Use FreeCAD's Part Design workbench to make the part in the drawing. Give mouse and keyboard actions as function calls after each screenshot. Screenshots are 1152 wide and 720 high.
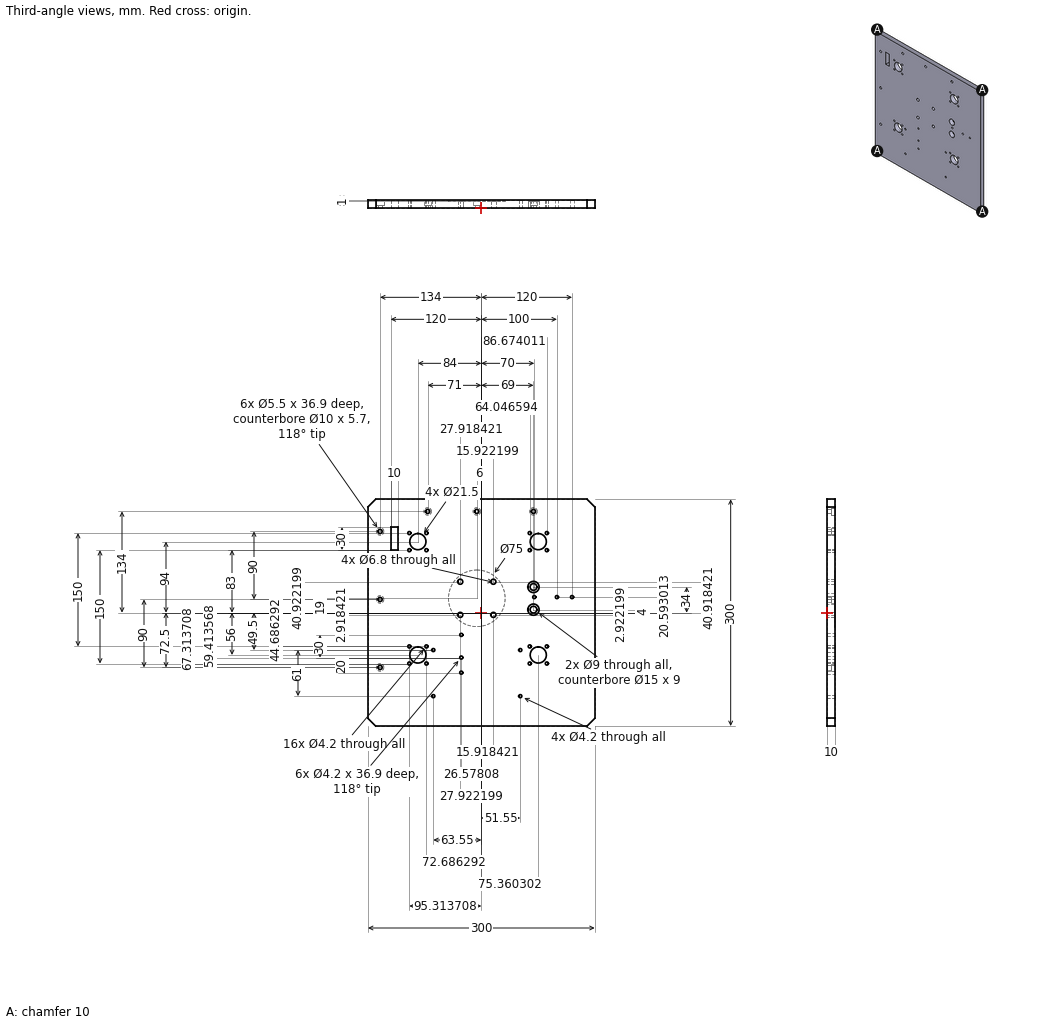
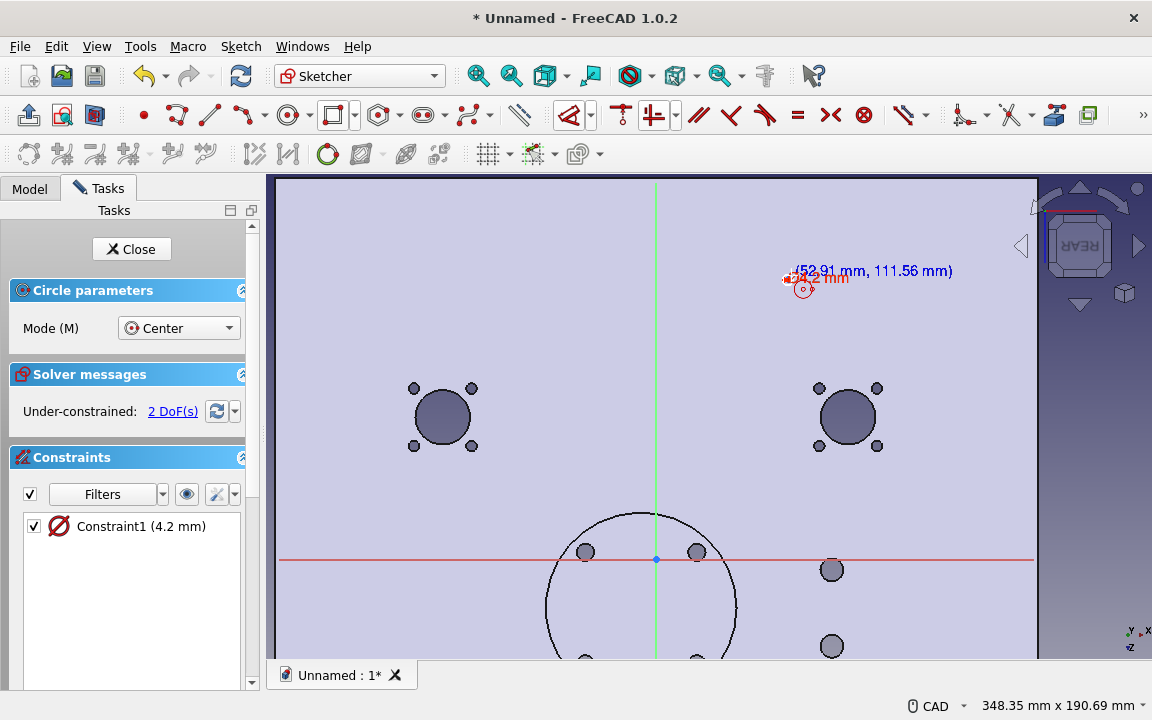
scroll(495, 279, up, 8)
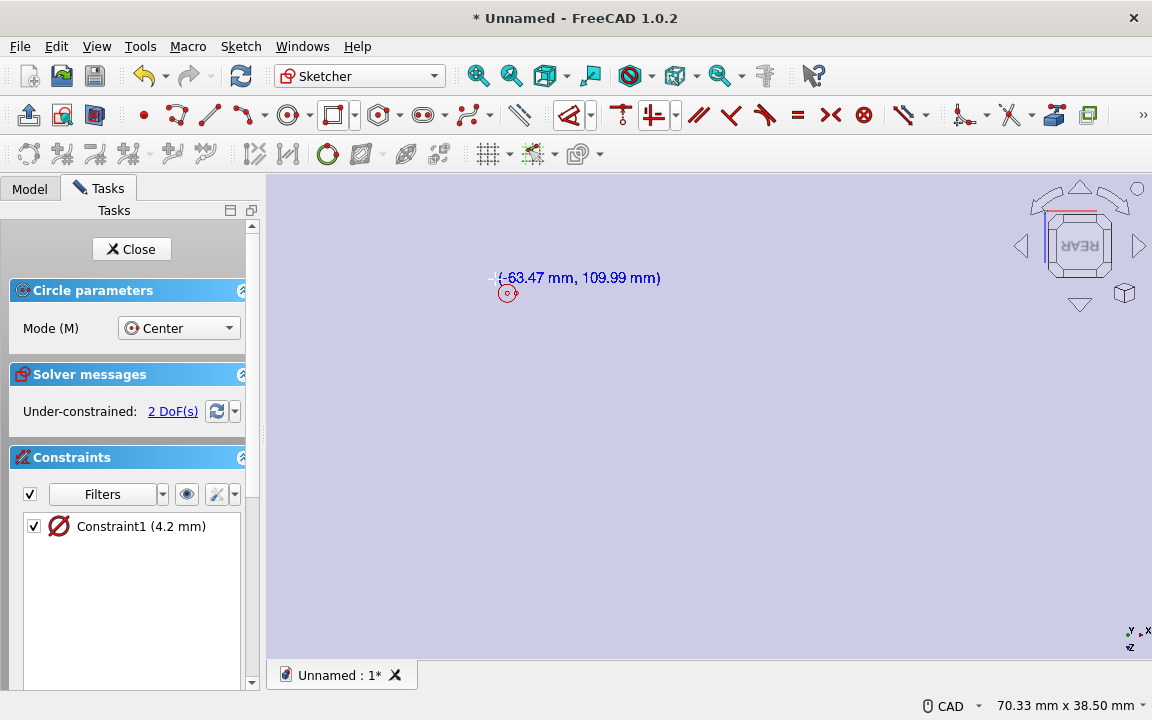
scroll(494, 279, down, 8)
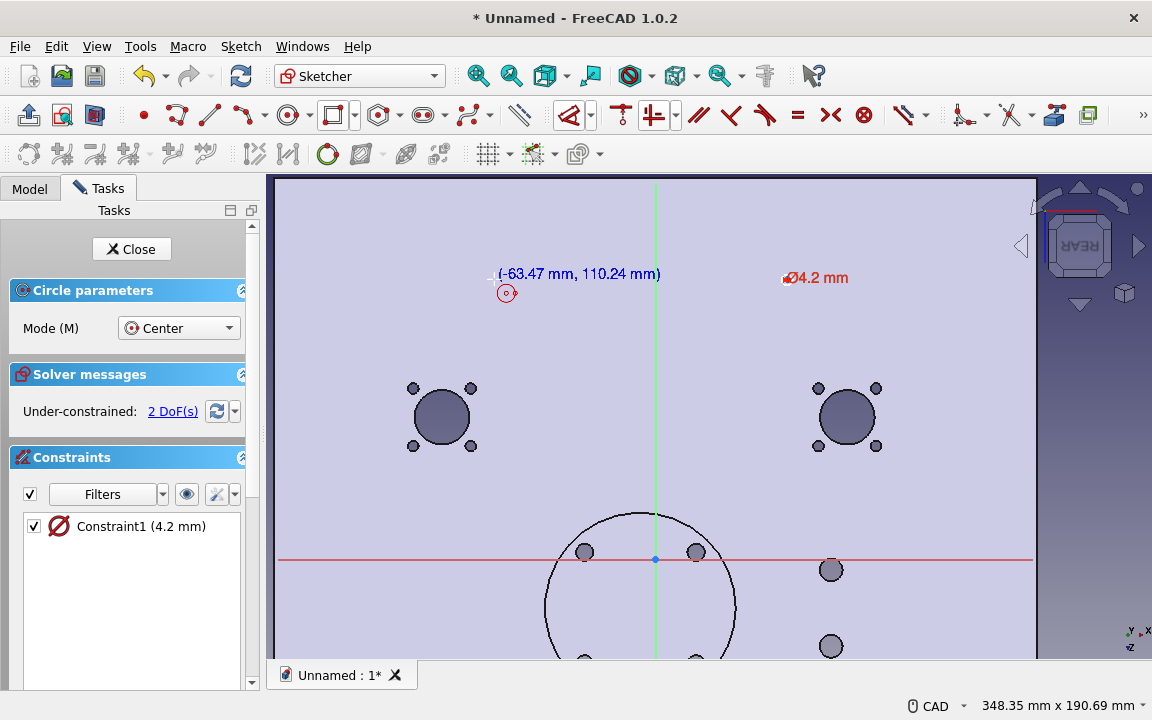
click(494, 279)
move(498, 275)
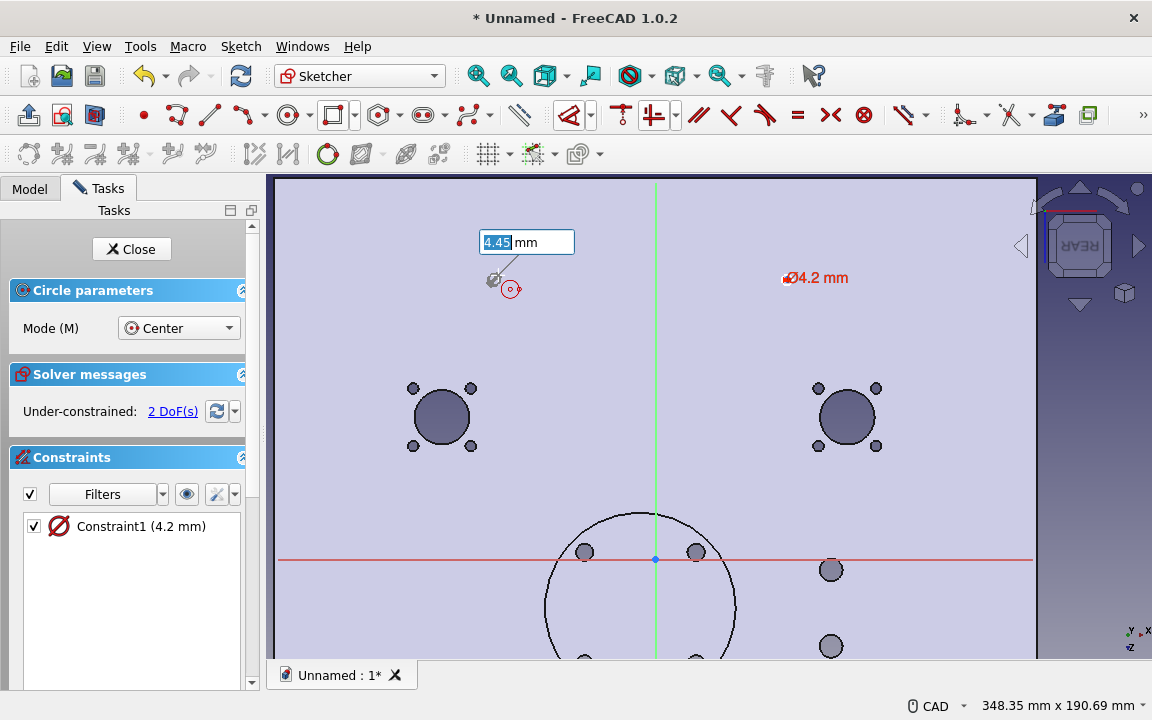
text(4.2)
key(Return)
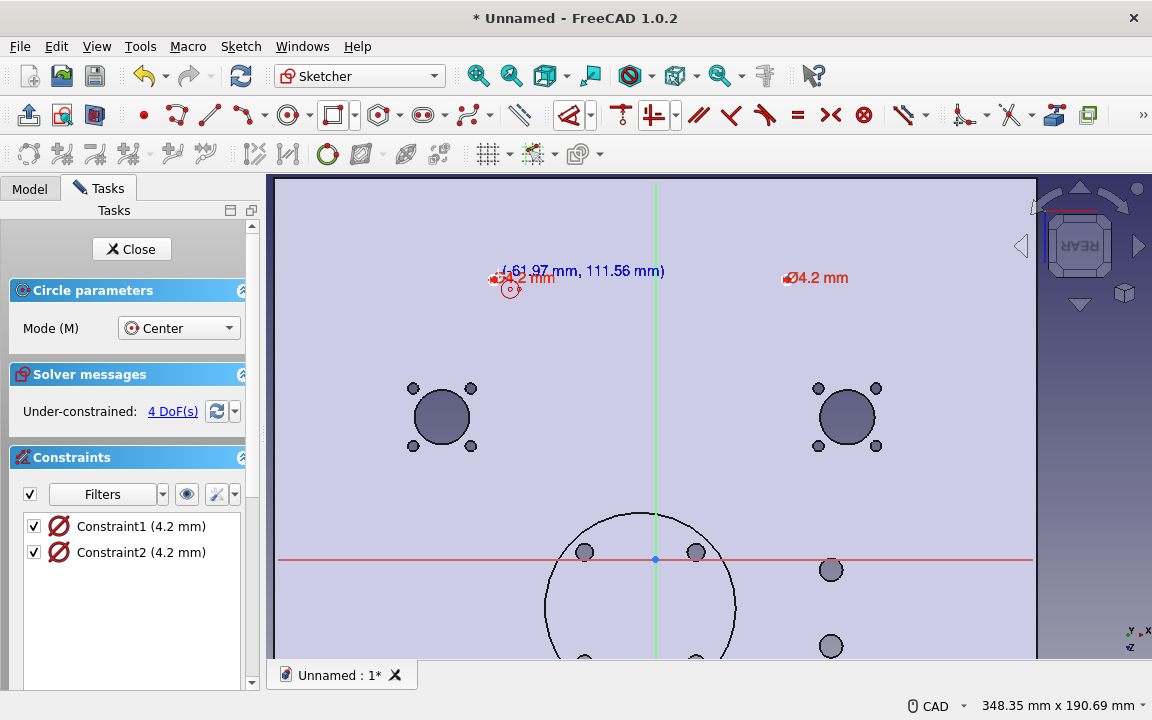
scroll(494, 434, up, 8)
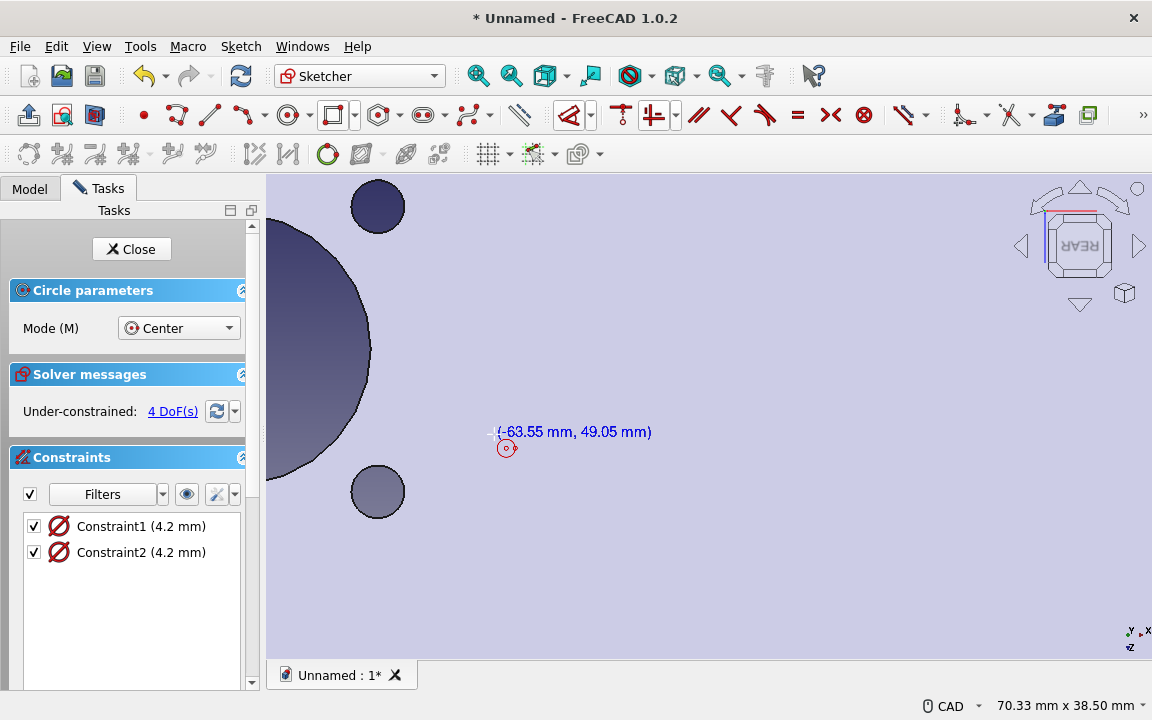
scroll(494, 434, down, 8)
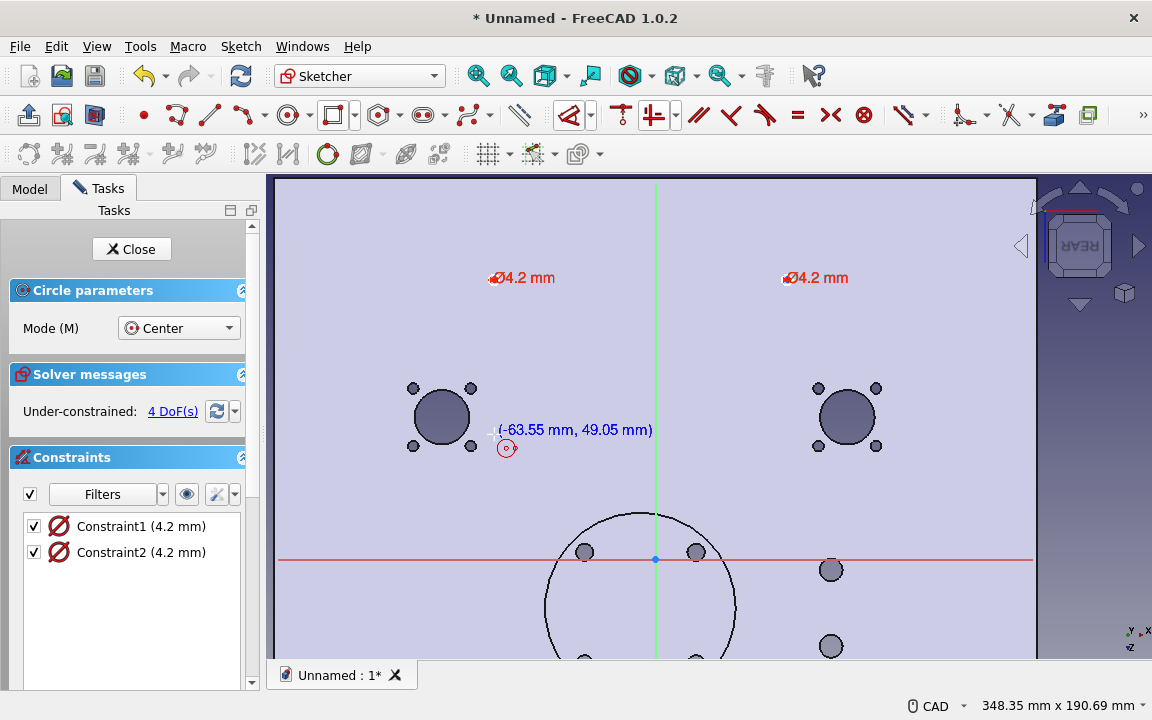
click(494, 434)
move(498, 430)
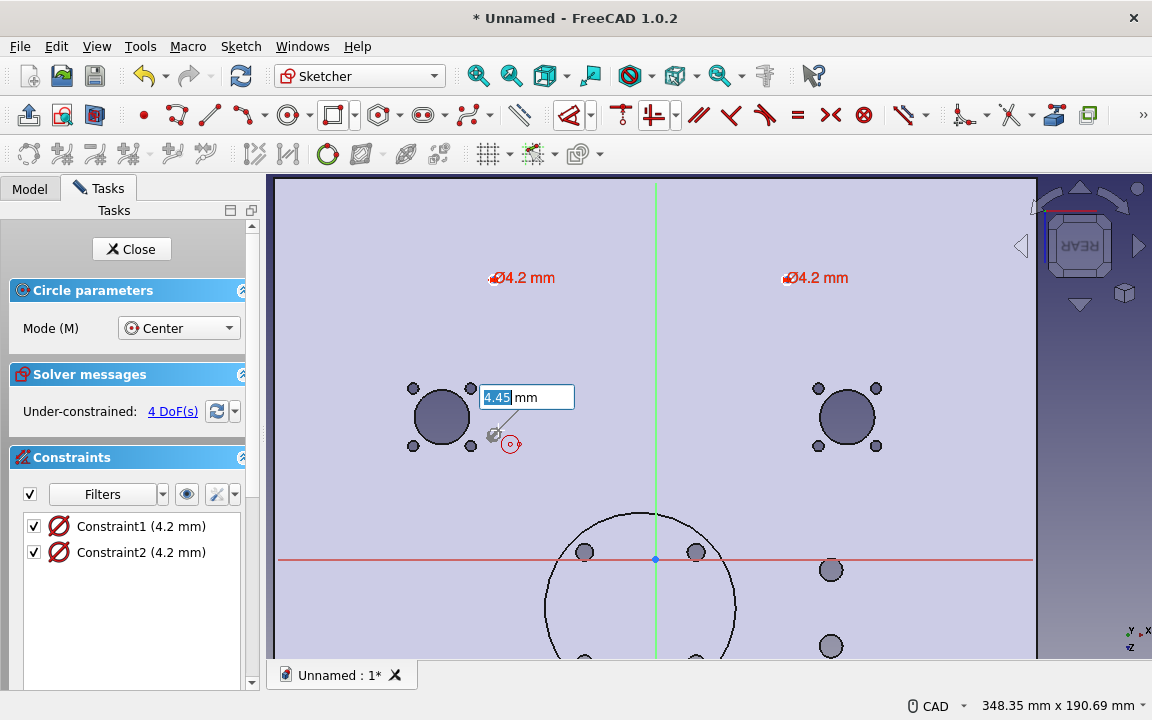
text(4.2)
key(Return)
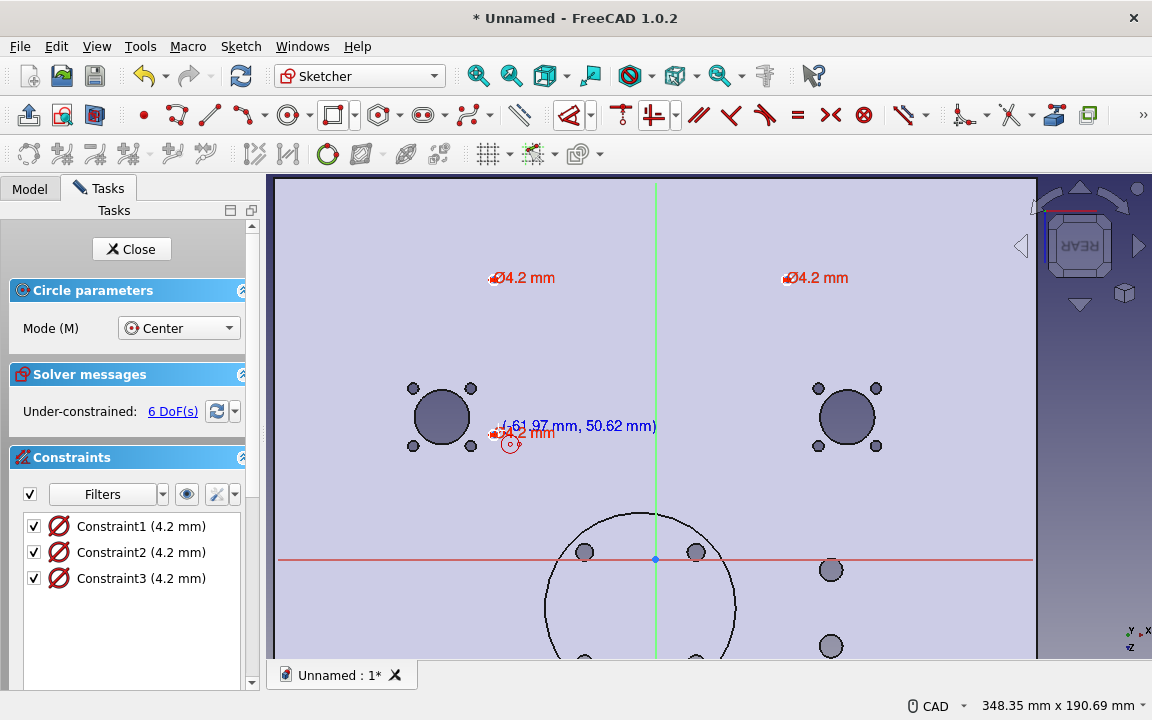
scroll(787, 434, up, 8)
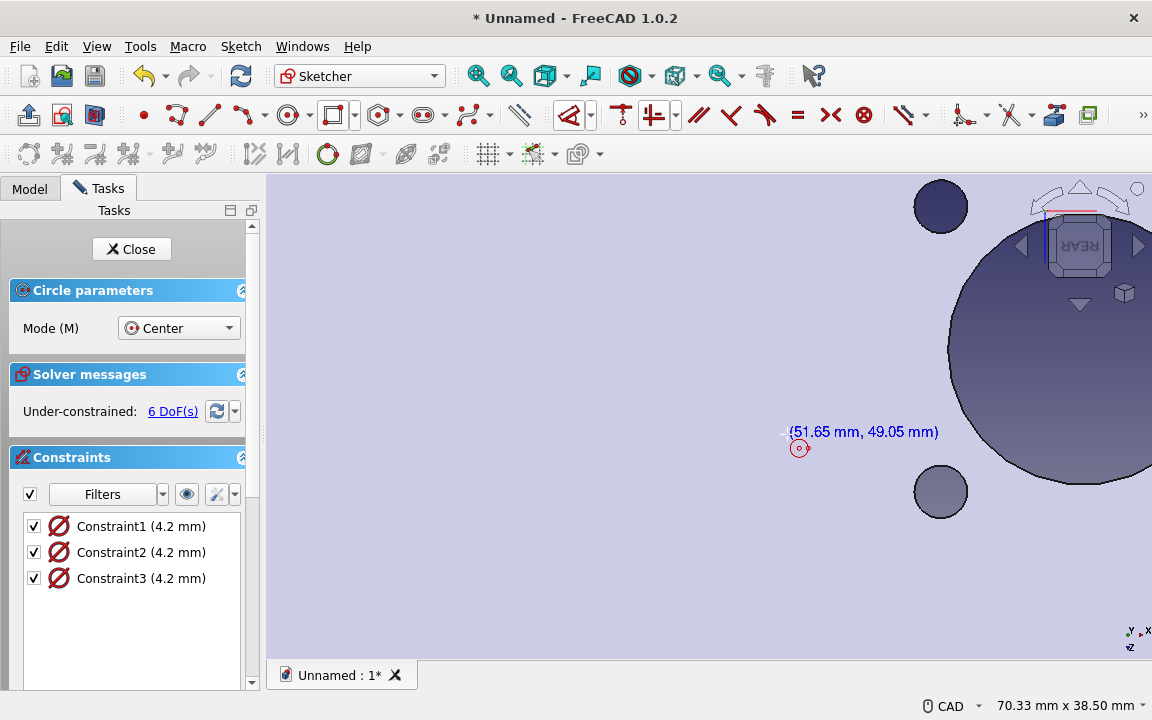
scroll(788, 434, down, 8)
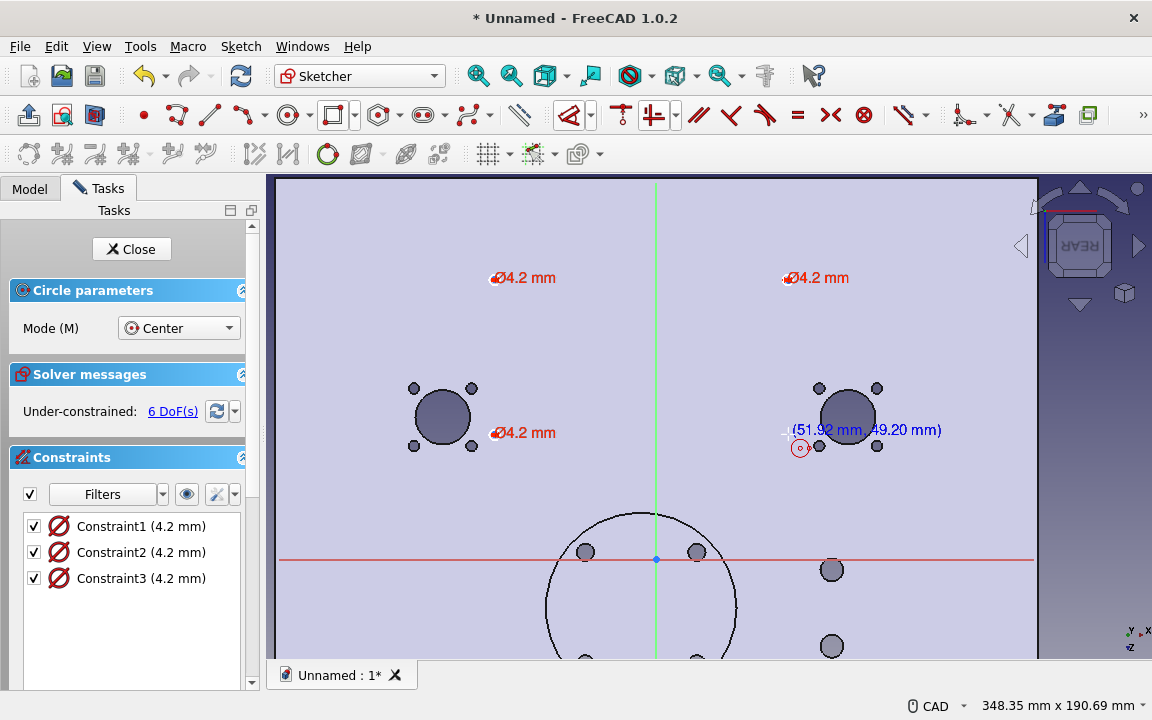
click(788, 434)
move(791, 430)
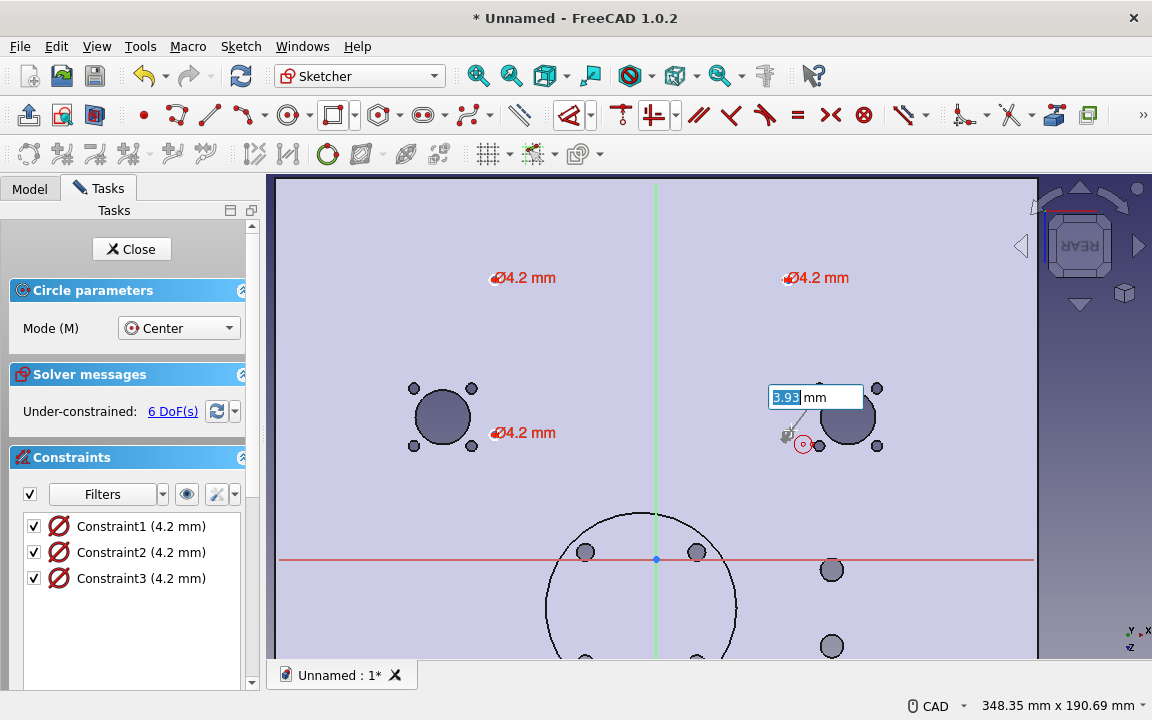
text(4.2)
key(Return)
key(Escape)